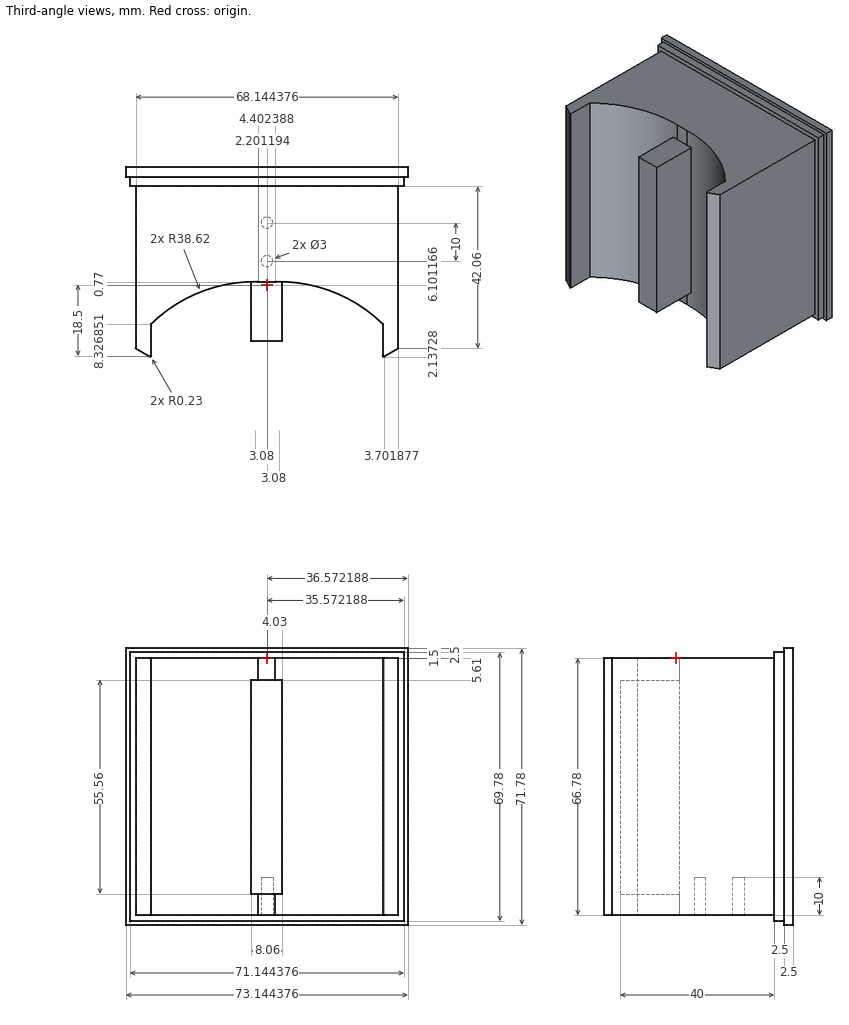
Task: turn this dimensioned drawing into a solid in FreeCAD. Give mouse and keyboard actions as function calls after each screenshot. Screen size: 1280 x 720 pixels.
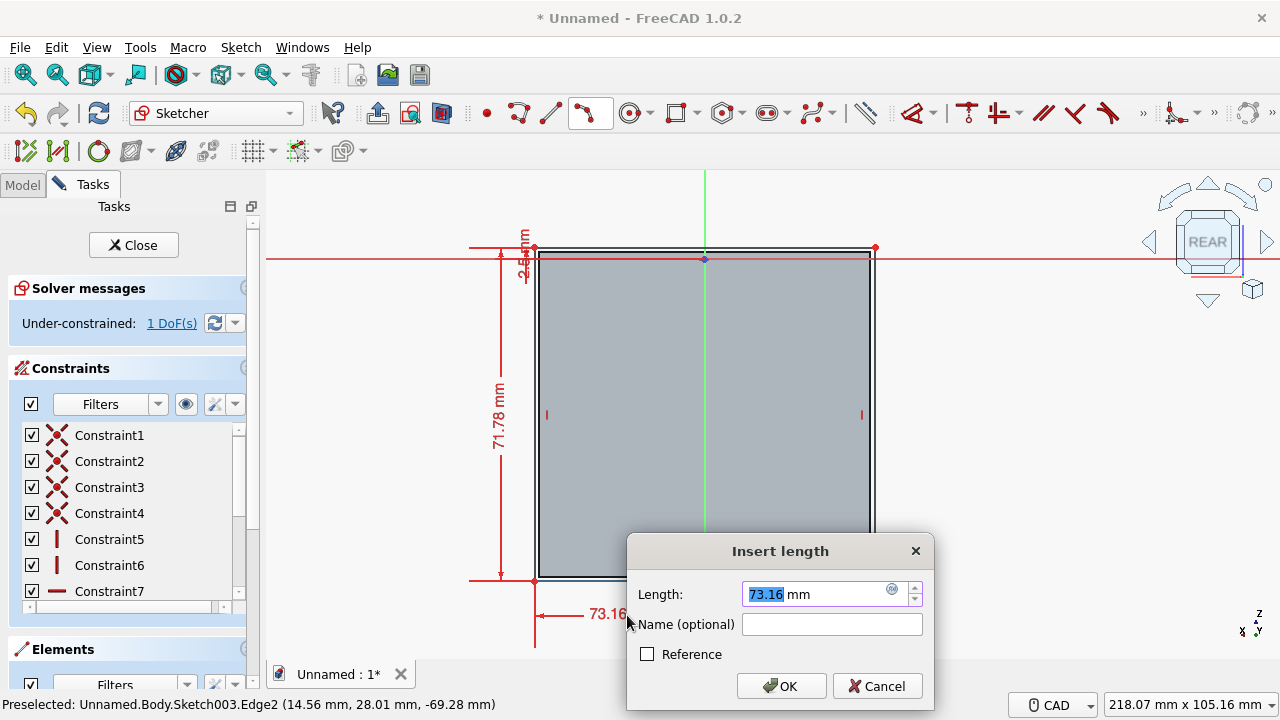
text(73.144376)
key(Return)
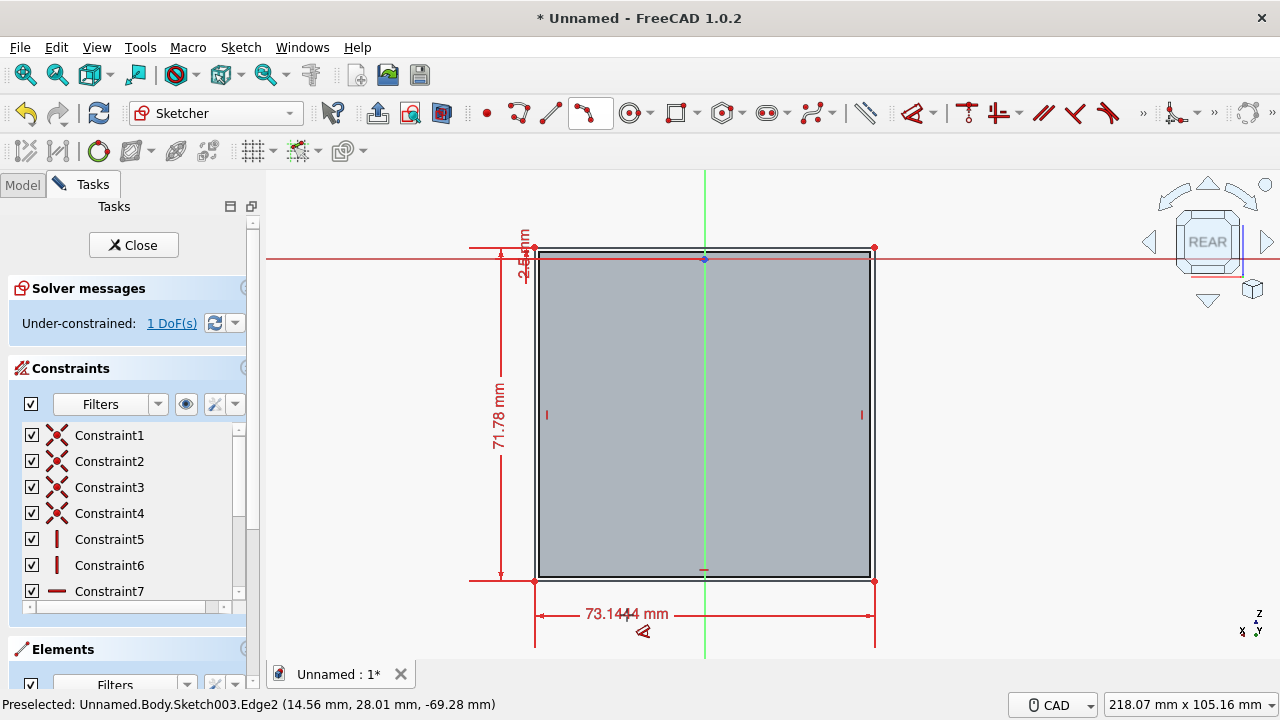
click(535, 248)
click(620, 214)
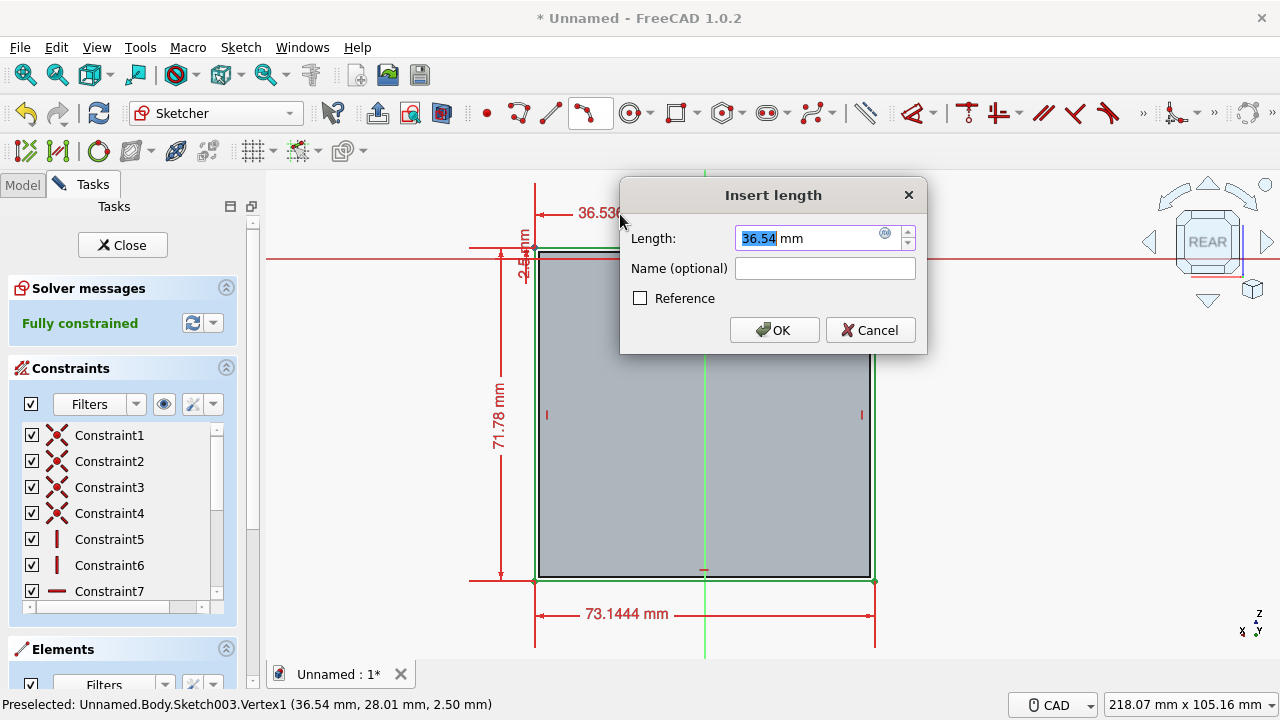
text(36.572188)
key(Return)
key(Escape)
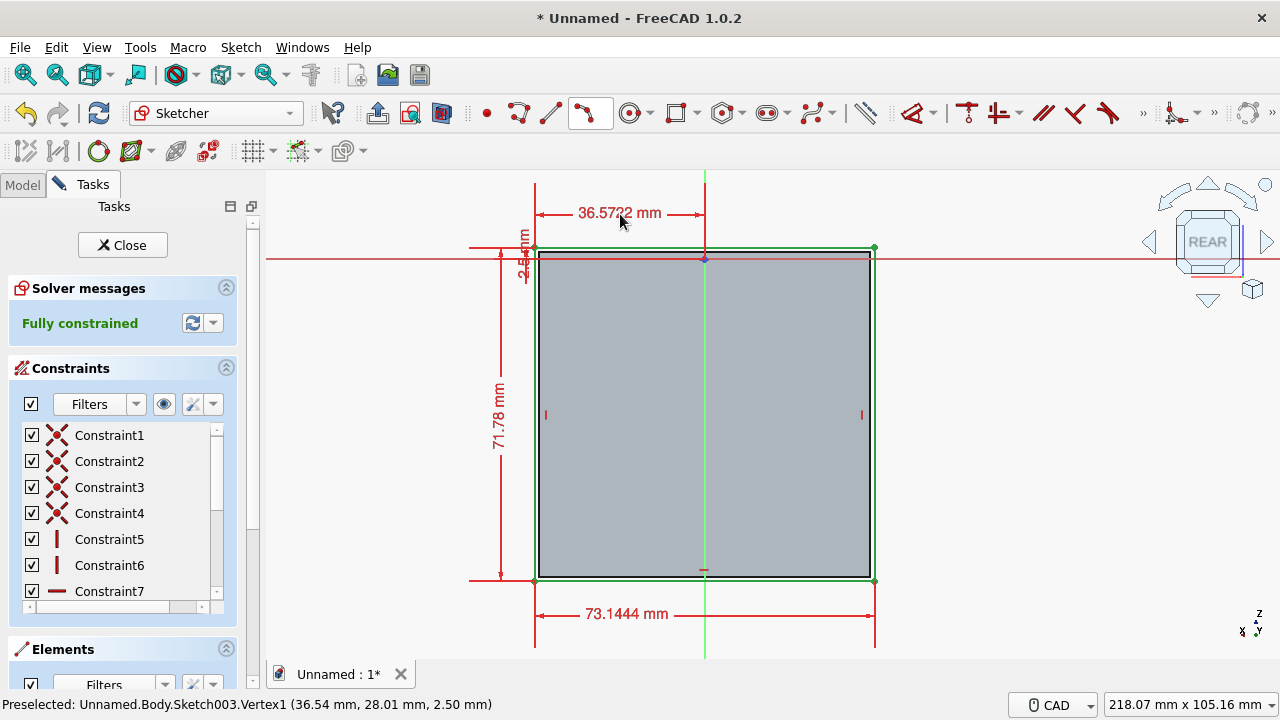
click(123, 245)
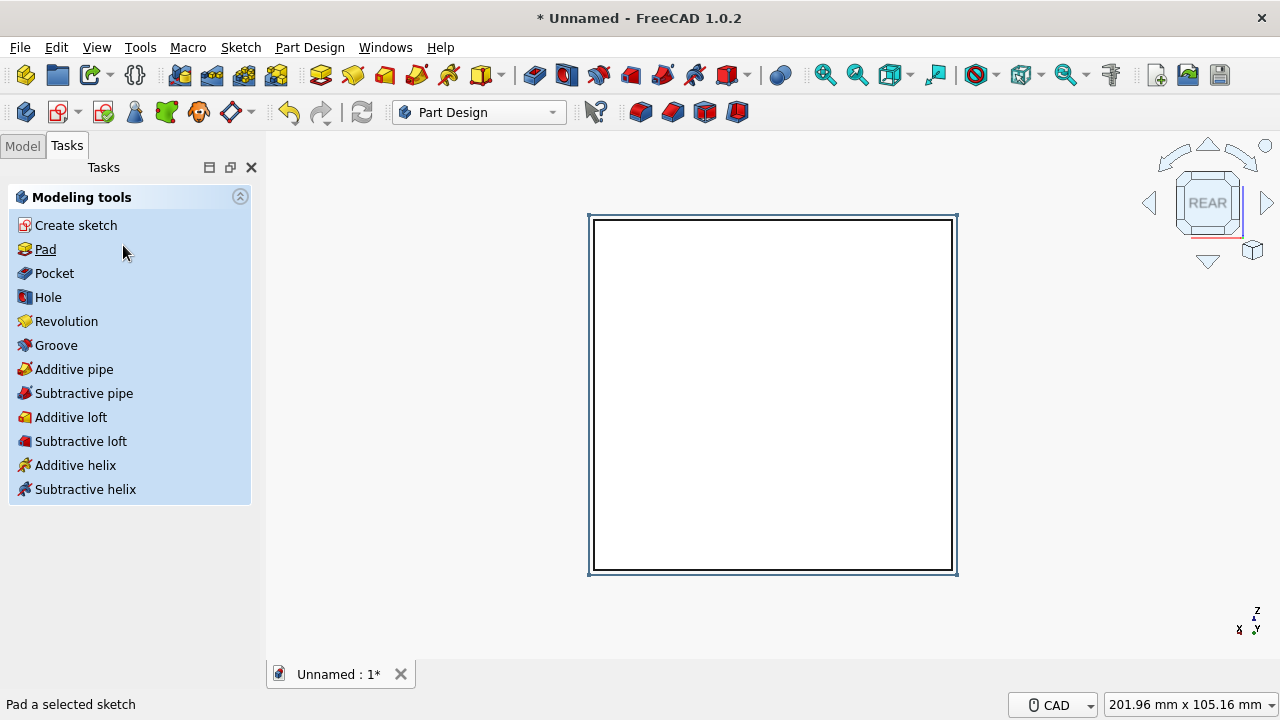
click(322, 76)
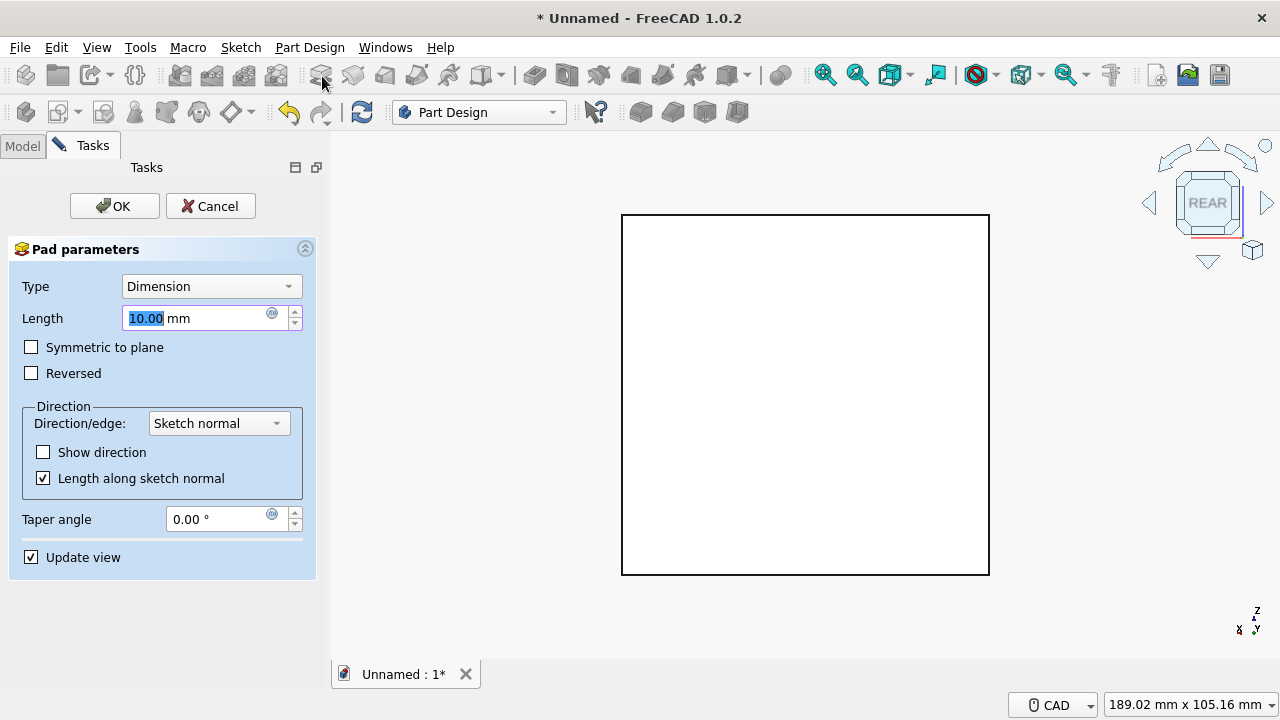
text(2.5)
key(Tab)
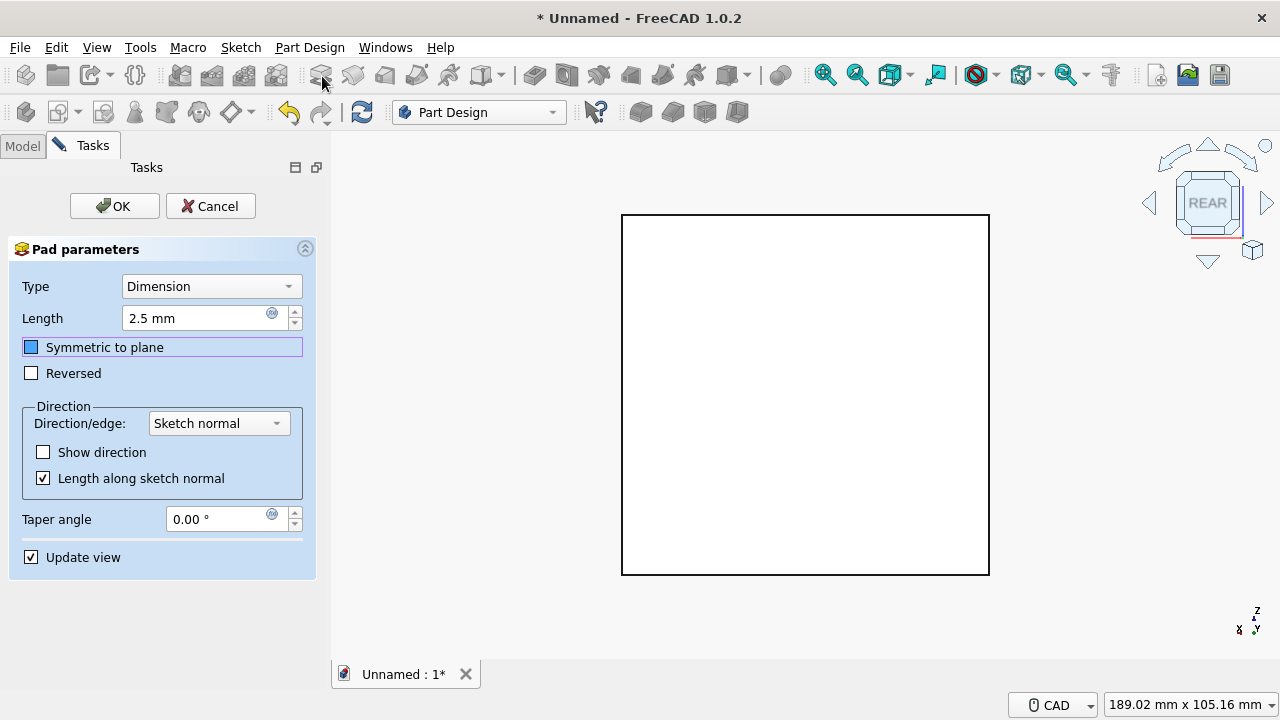
click(115, 206)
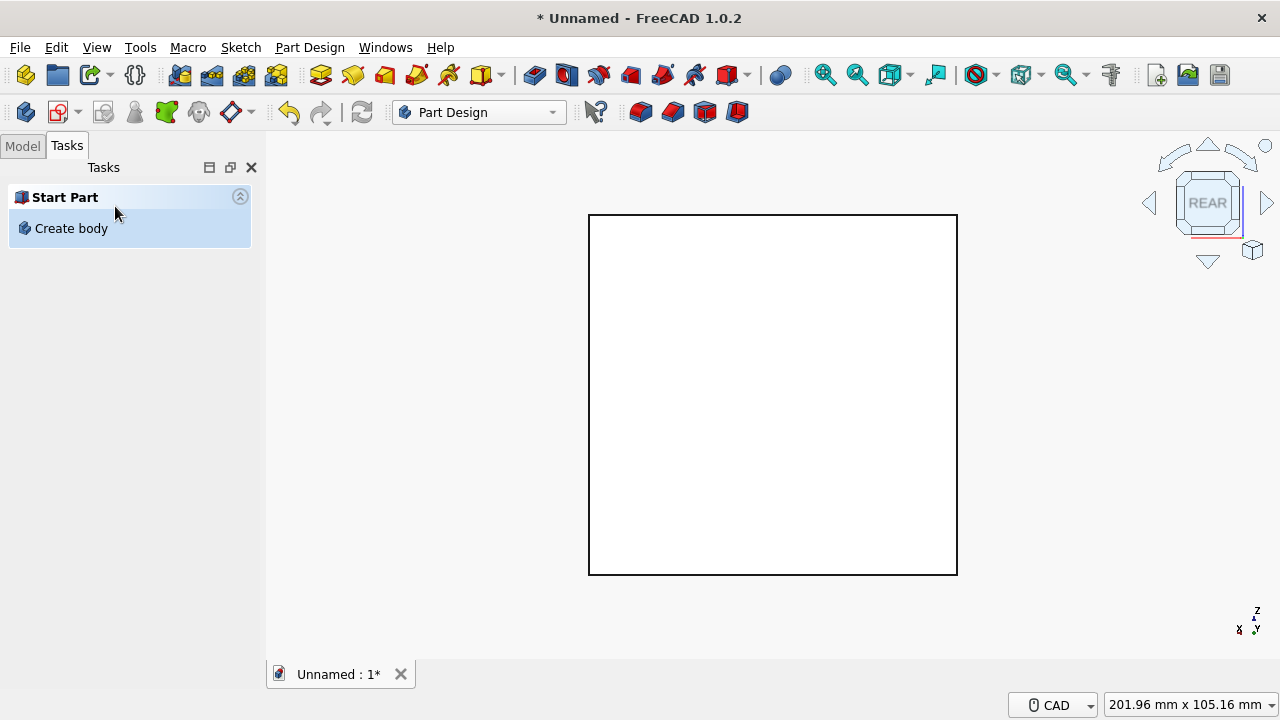
key(5)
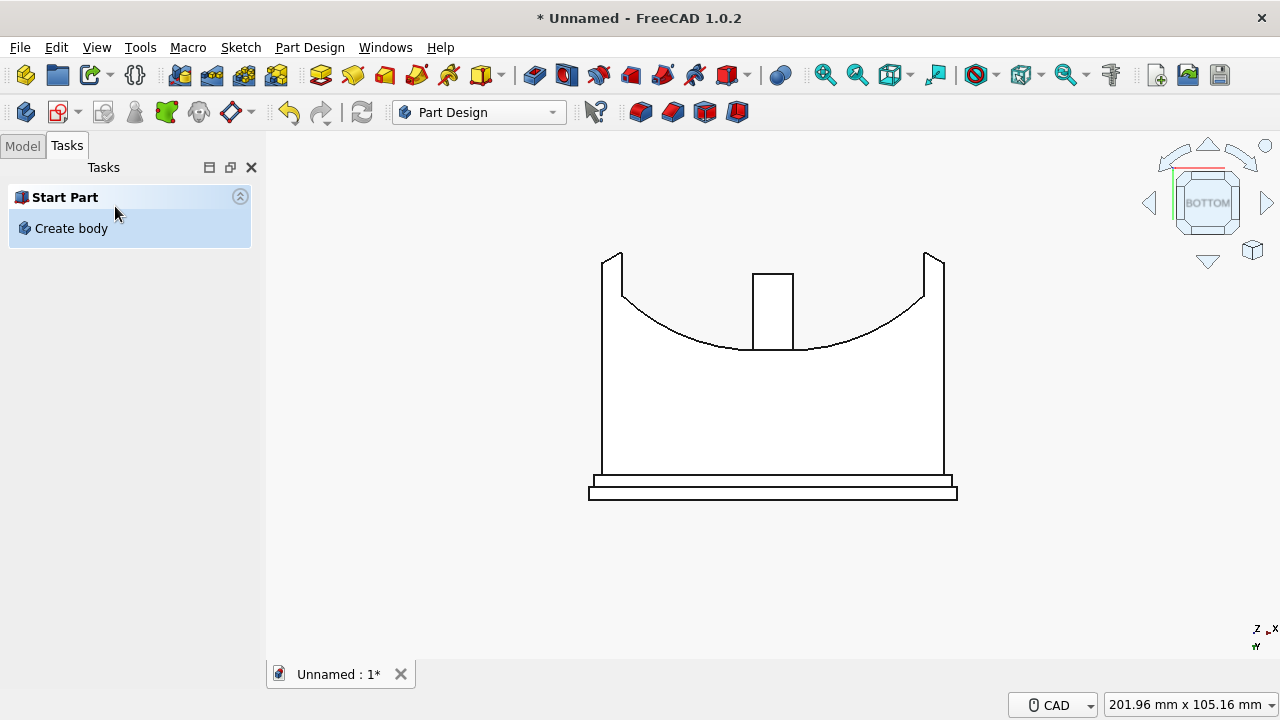
click(675, 394)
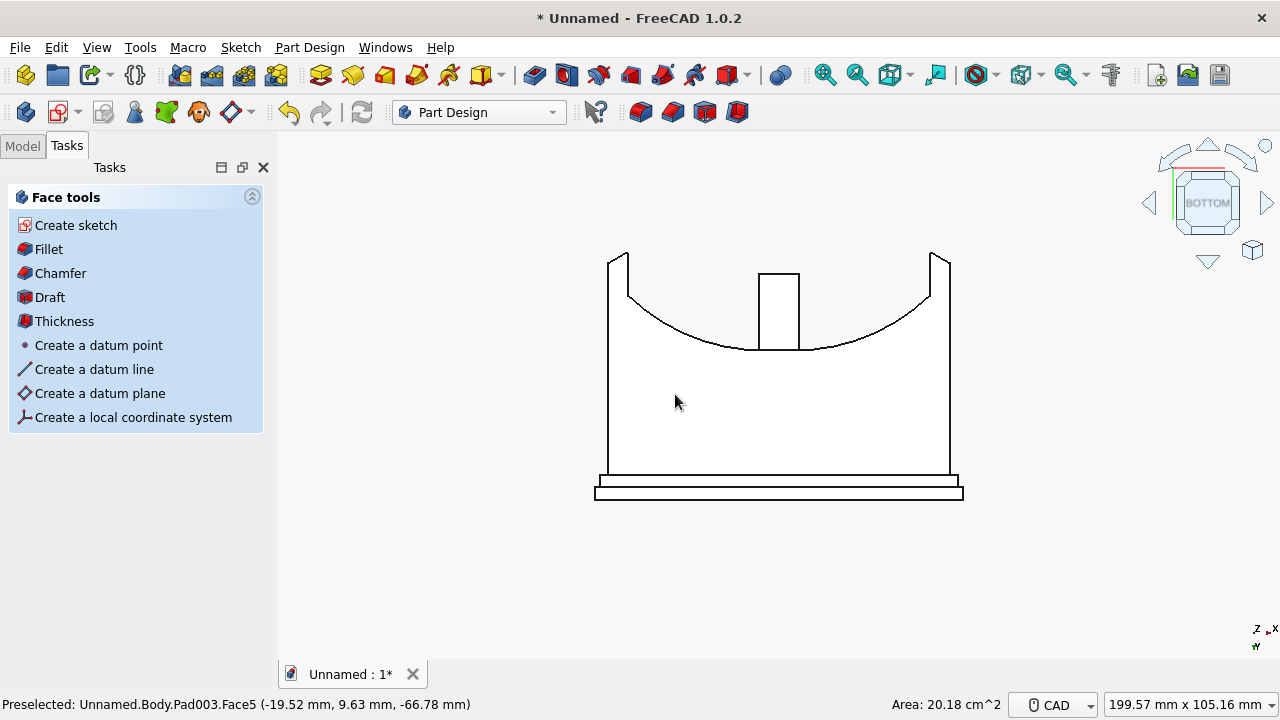
click(58, 112)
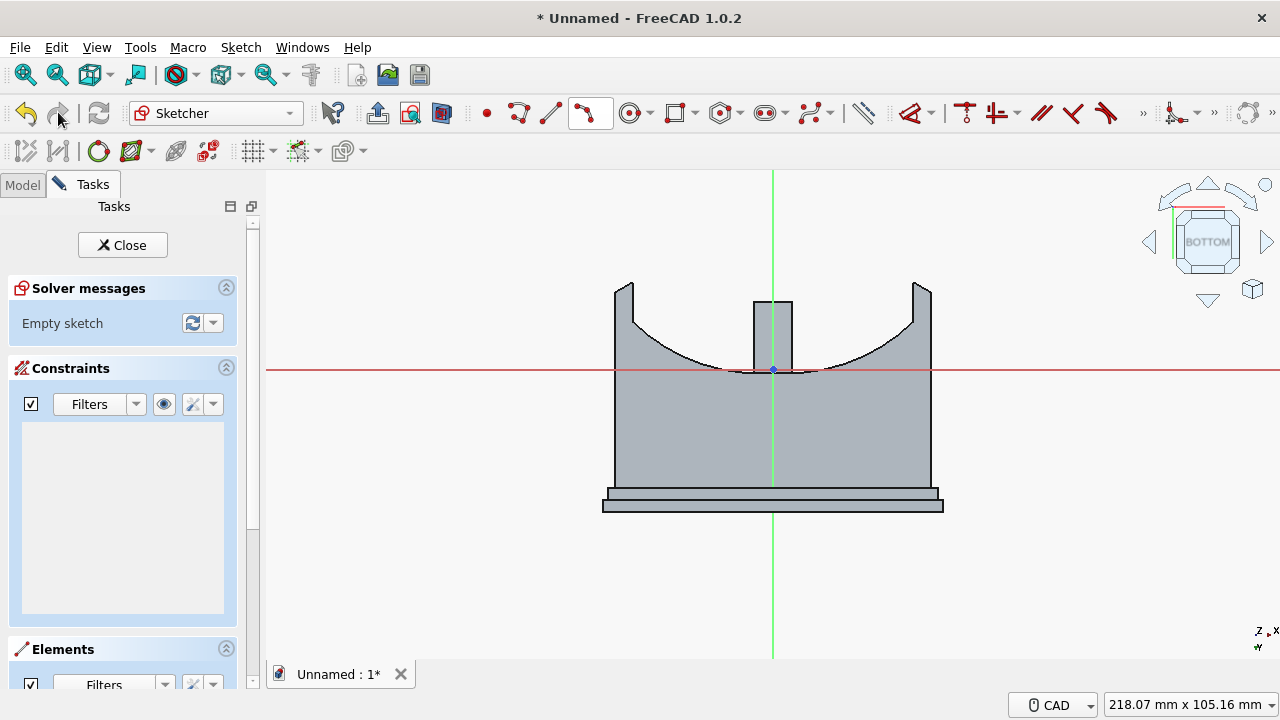
scroll(795, 409, up, 7)